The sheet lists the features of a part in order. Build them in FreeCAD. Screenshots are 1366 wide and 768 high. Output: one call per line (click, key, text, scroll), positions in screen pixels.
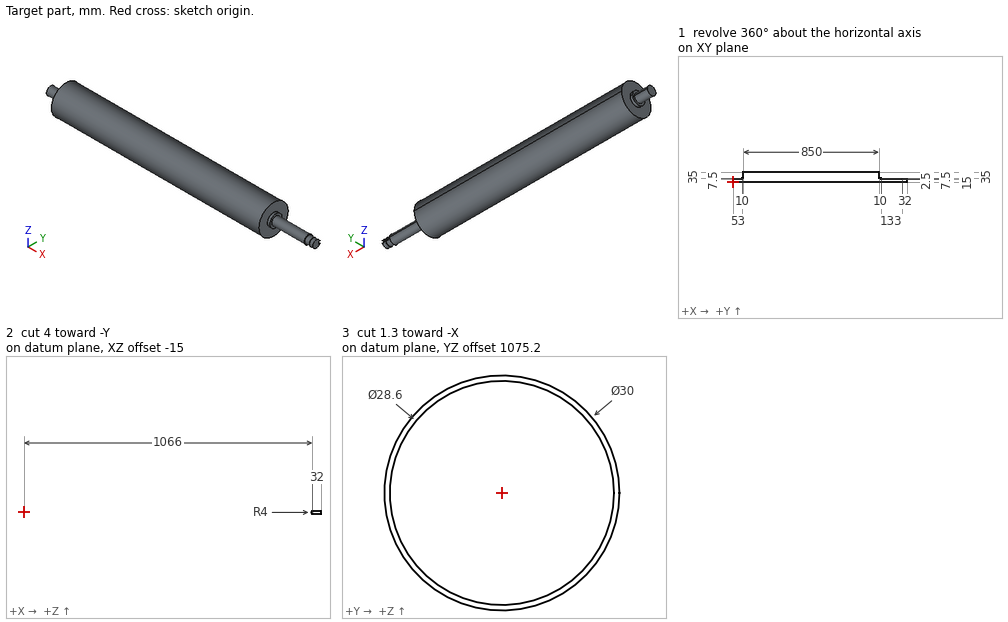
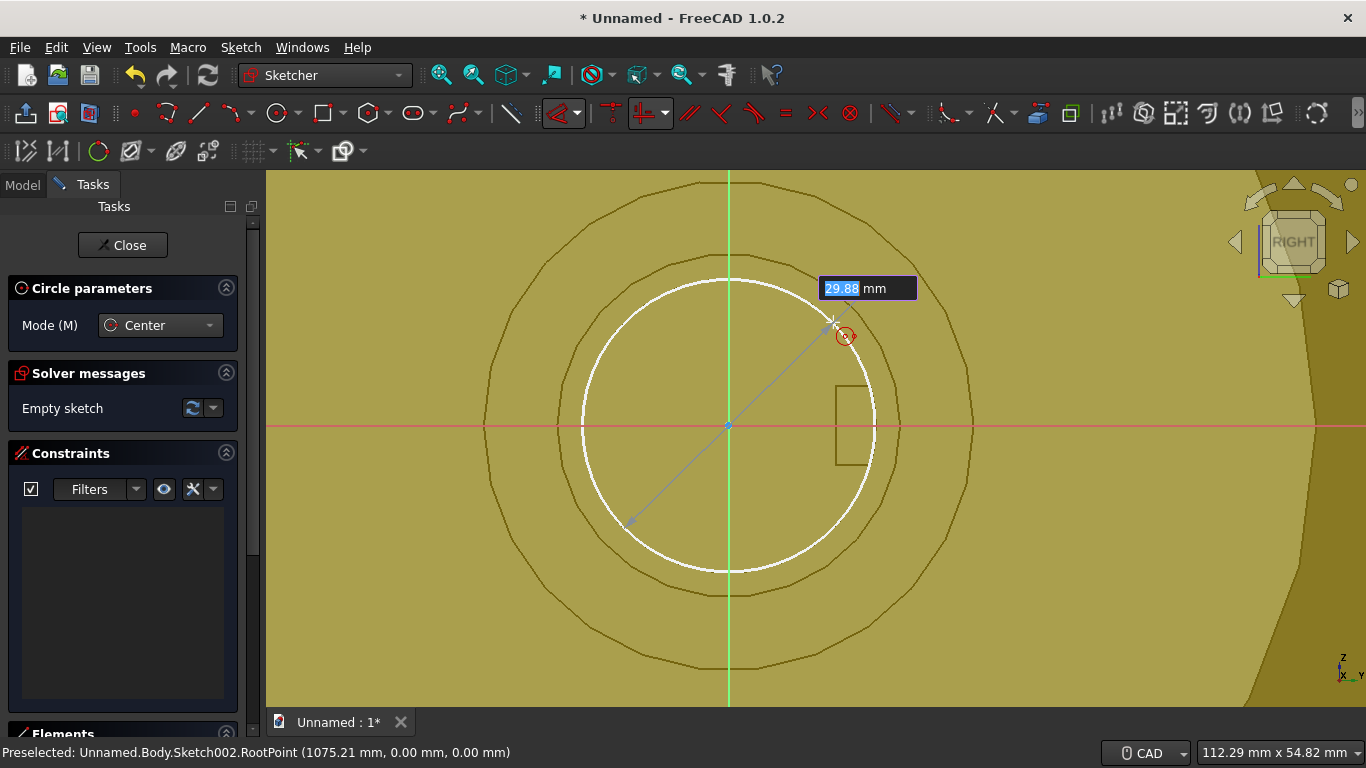
text(30)
key(Return)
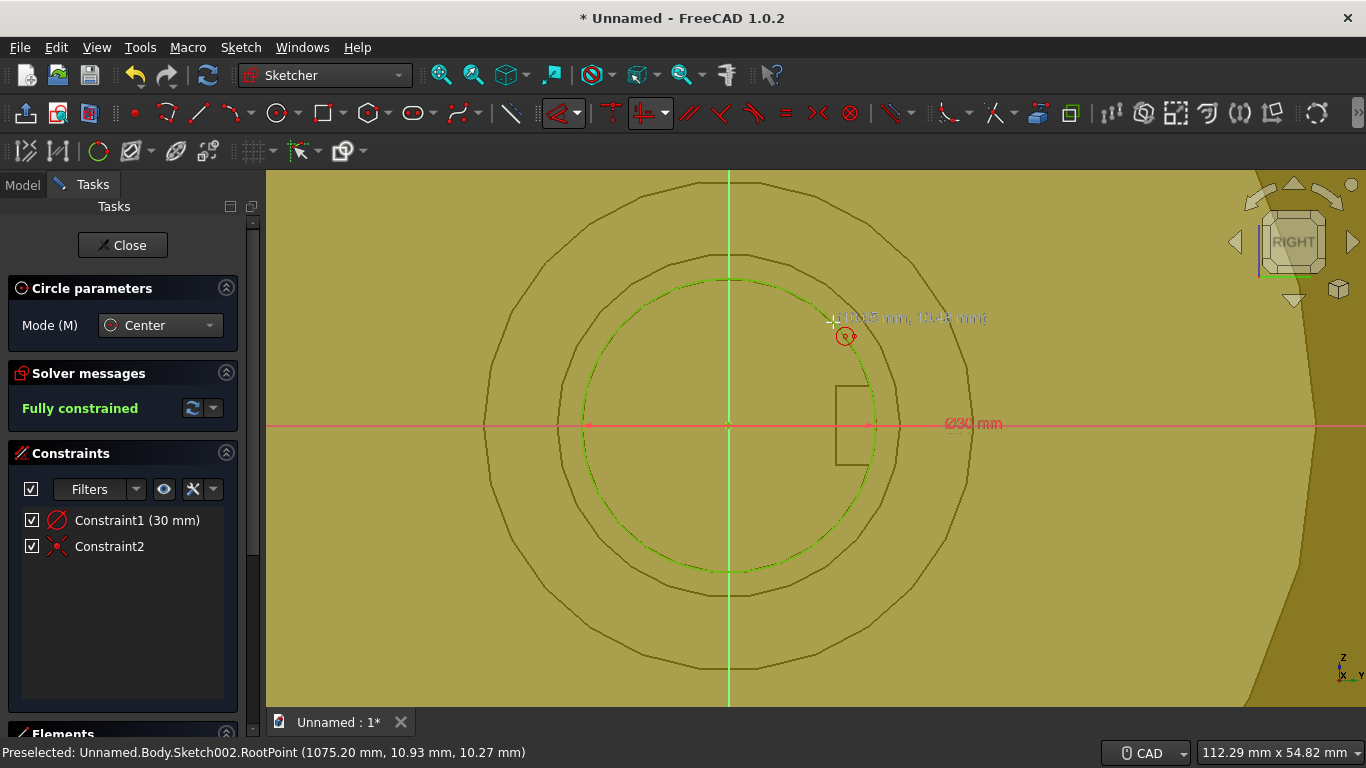
click(729, 426)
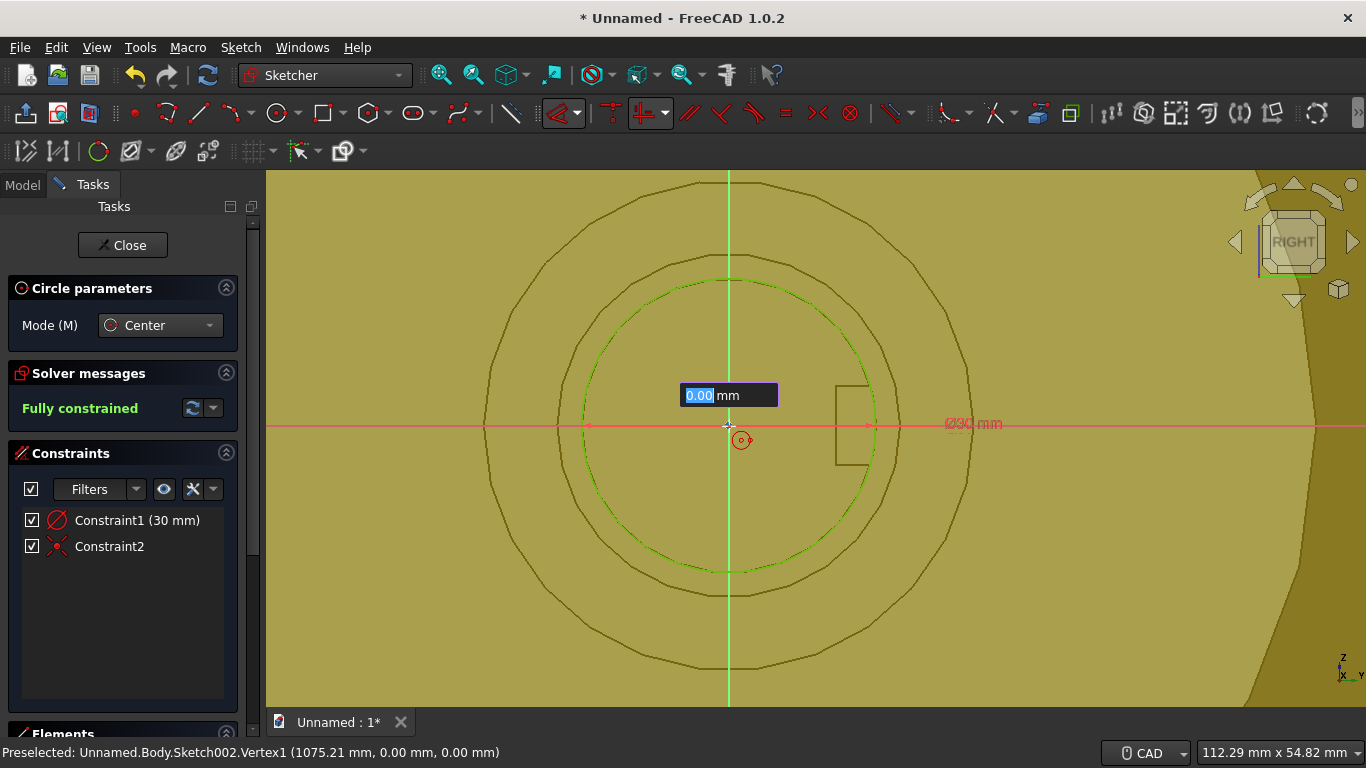
scroll(777, 294, up, 5)
move(775, 294)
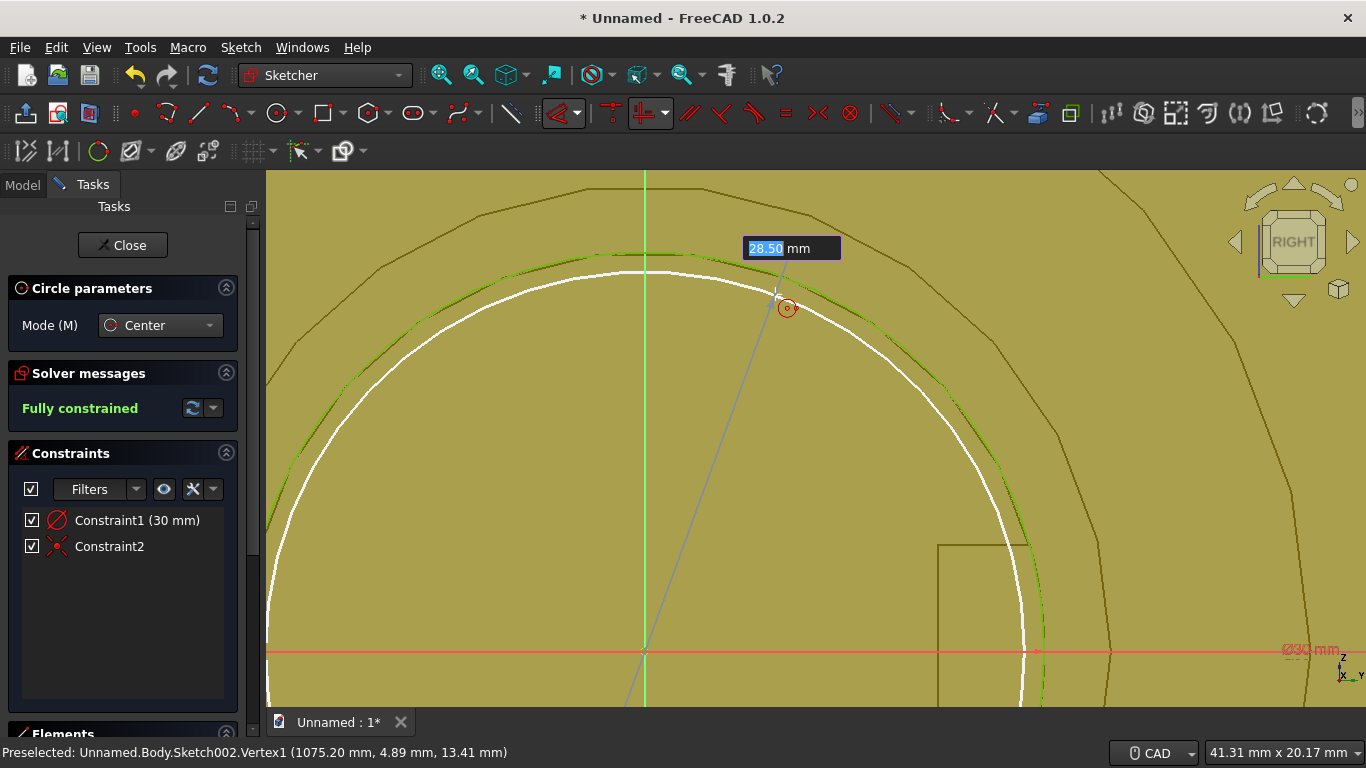
text(28.6)
key(Return)
key(Escape)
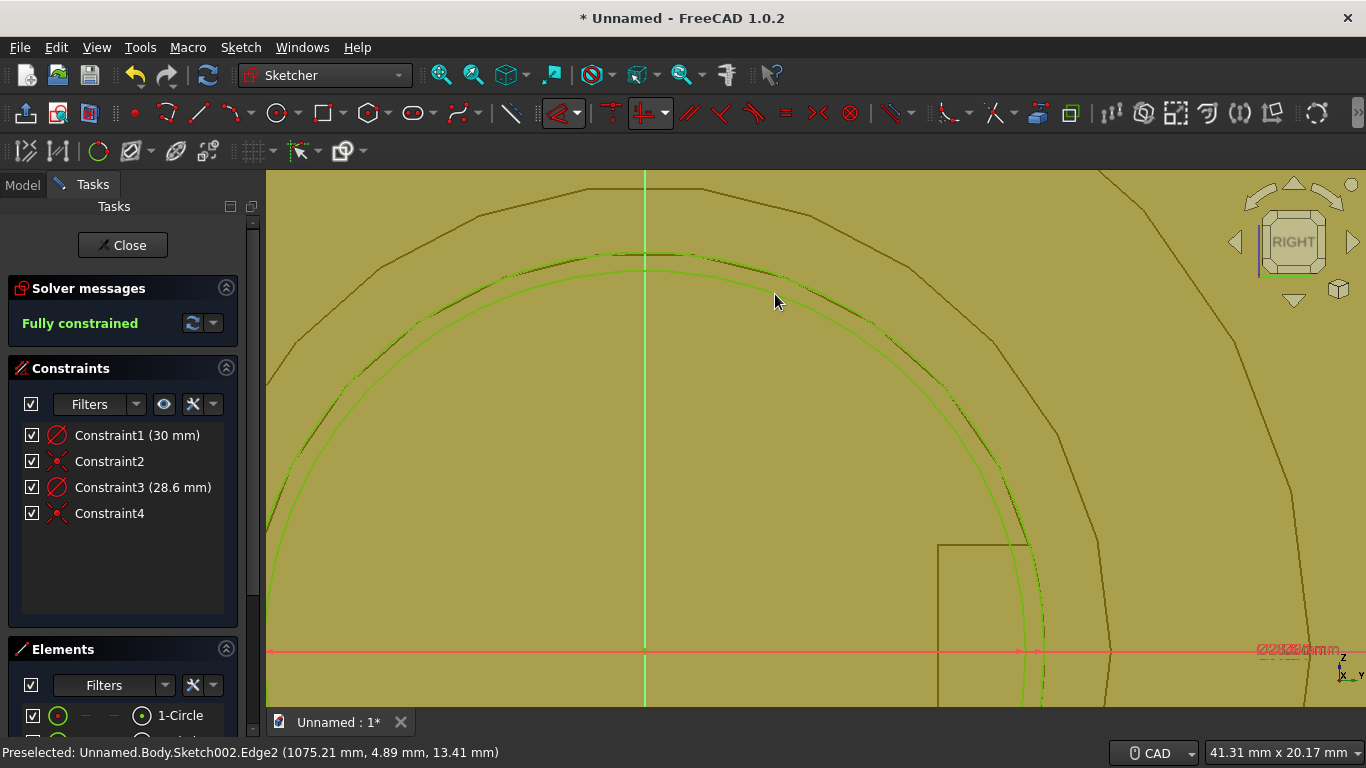
click(123, 245)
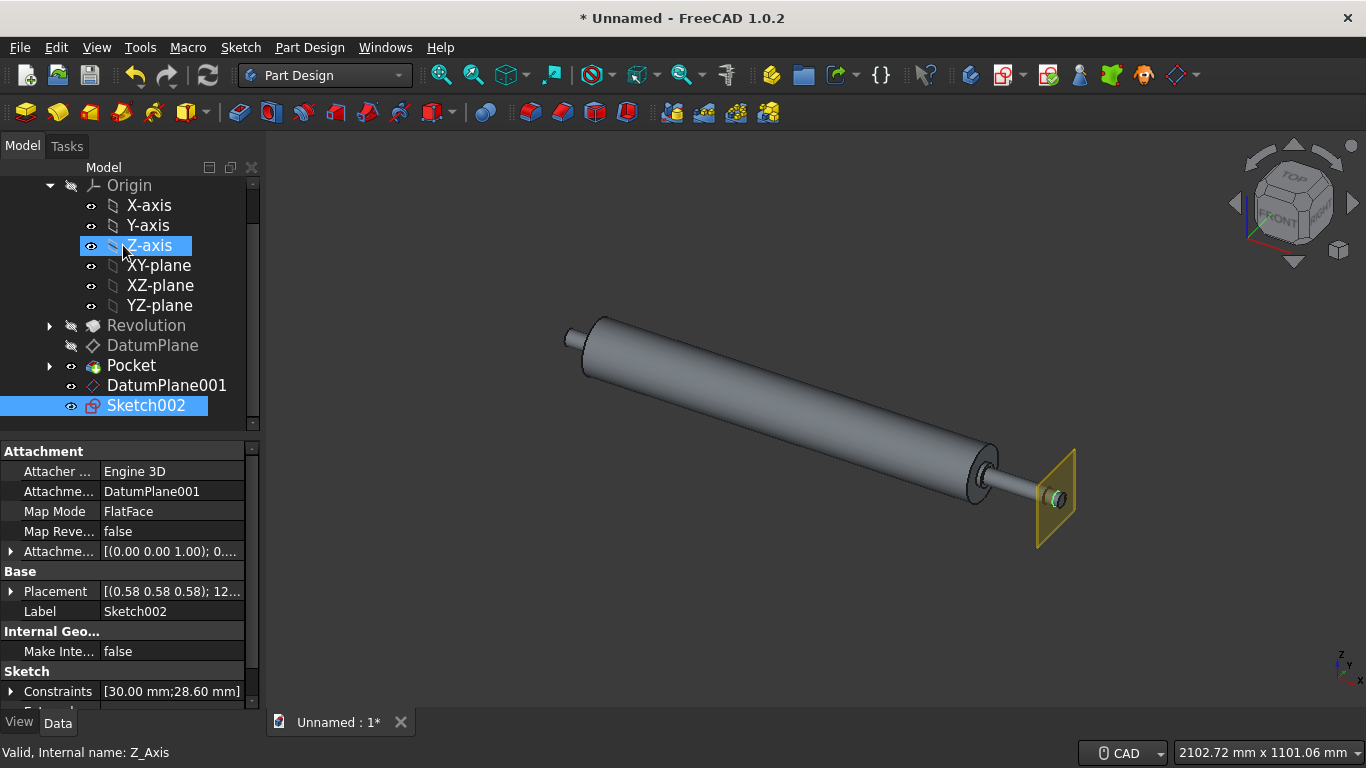
click(240, 112)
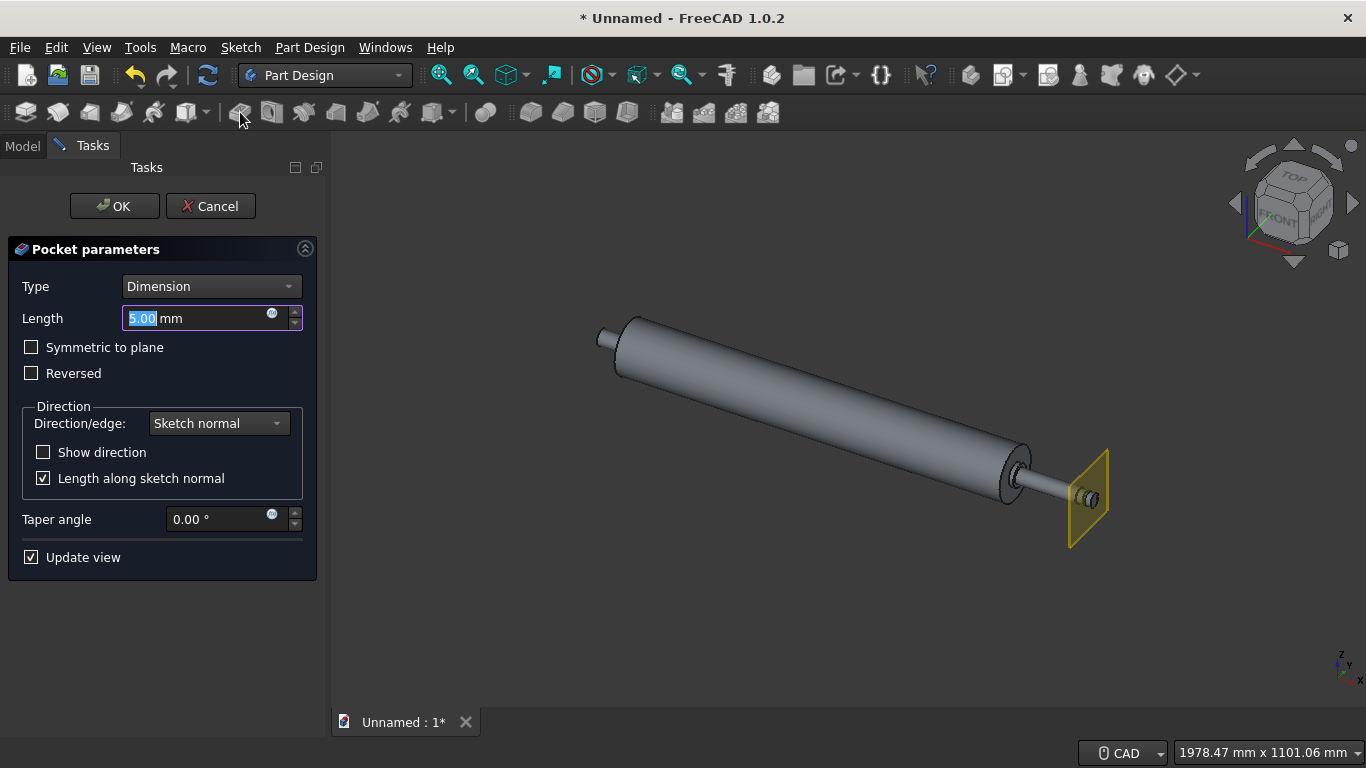
text(1.3)
key(Tab)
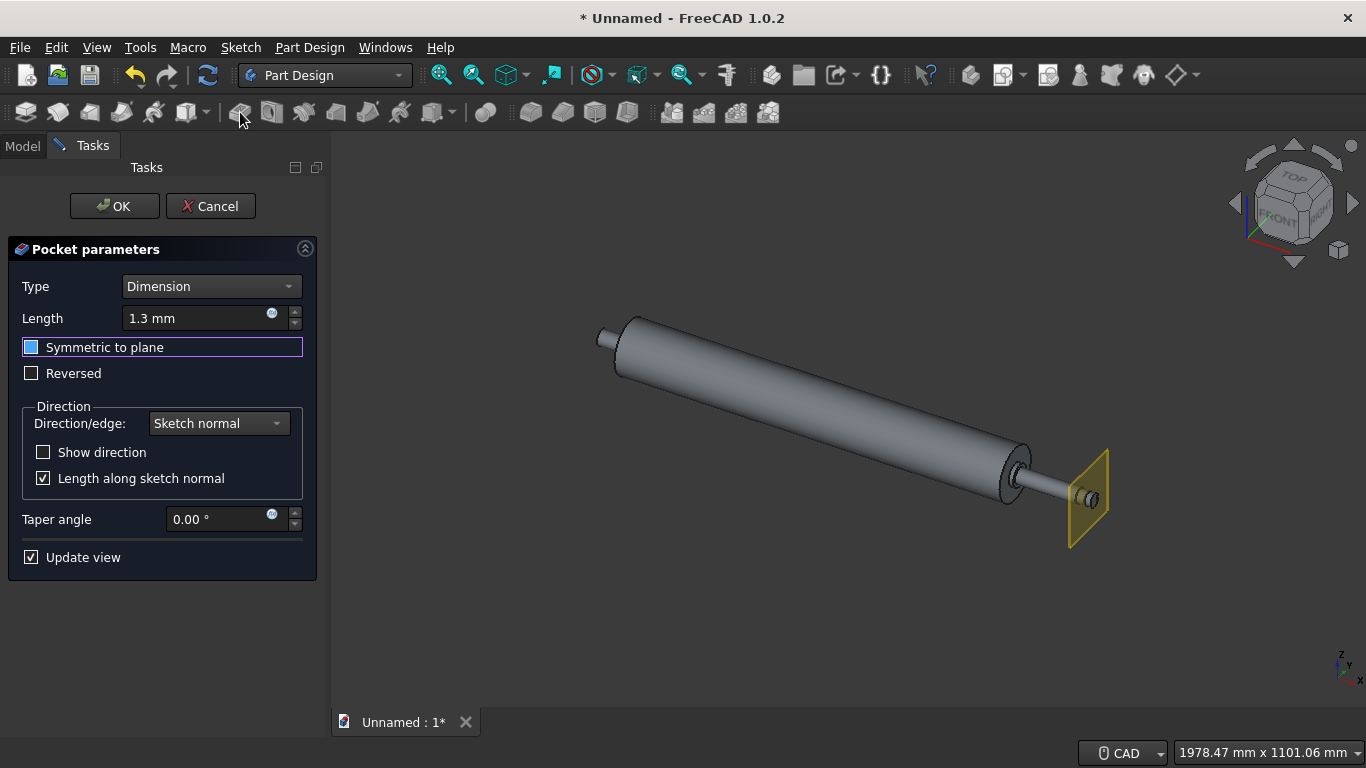
click(115, 206)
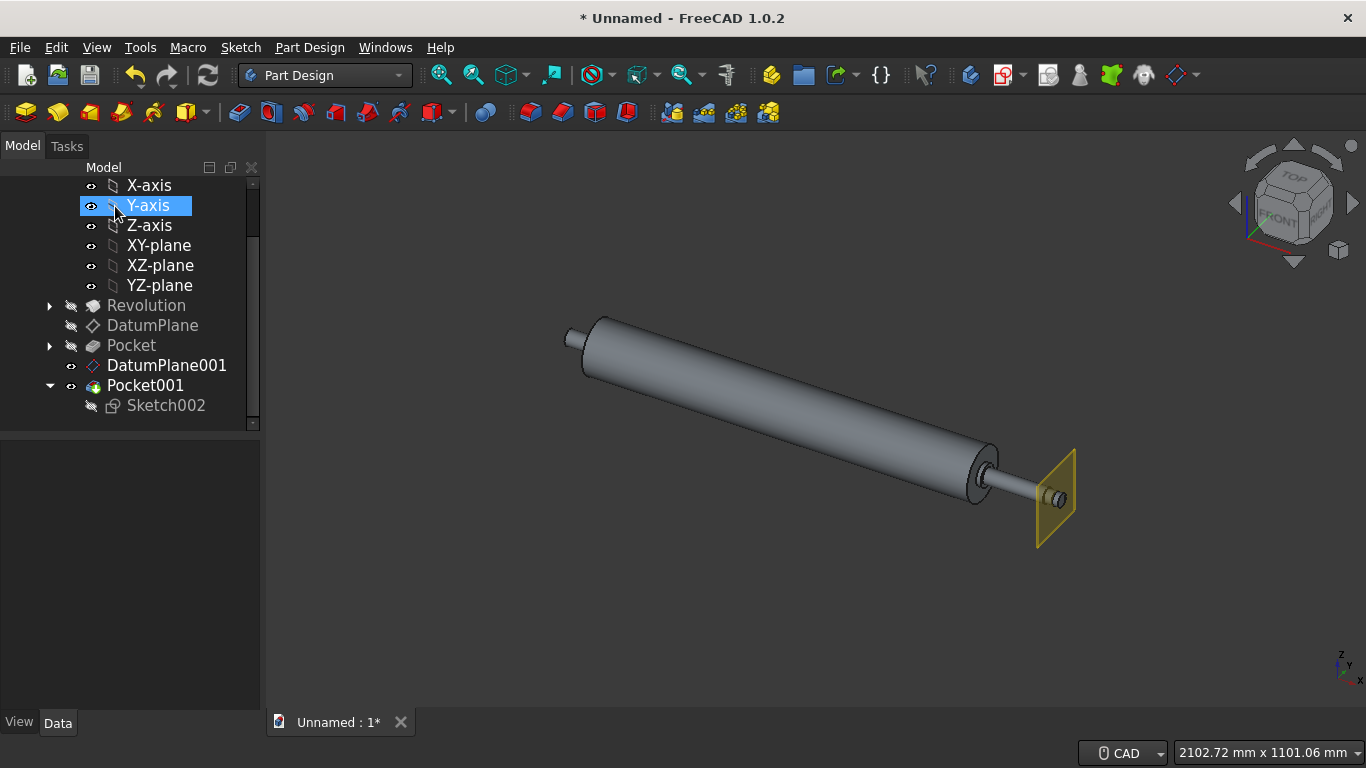
click(116, 366)
key(space)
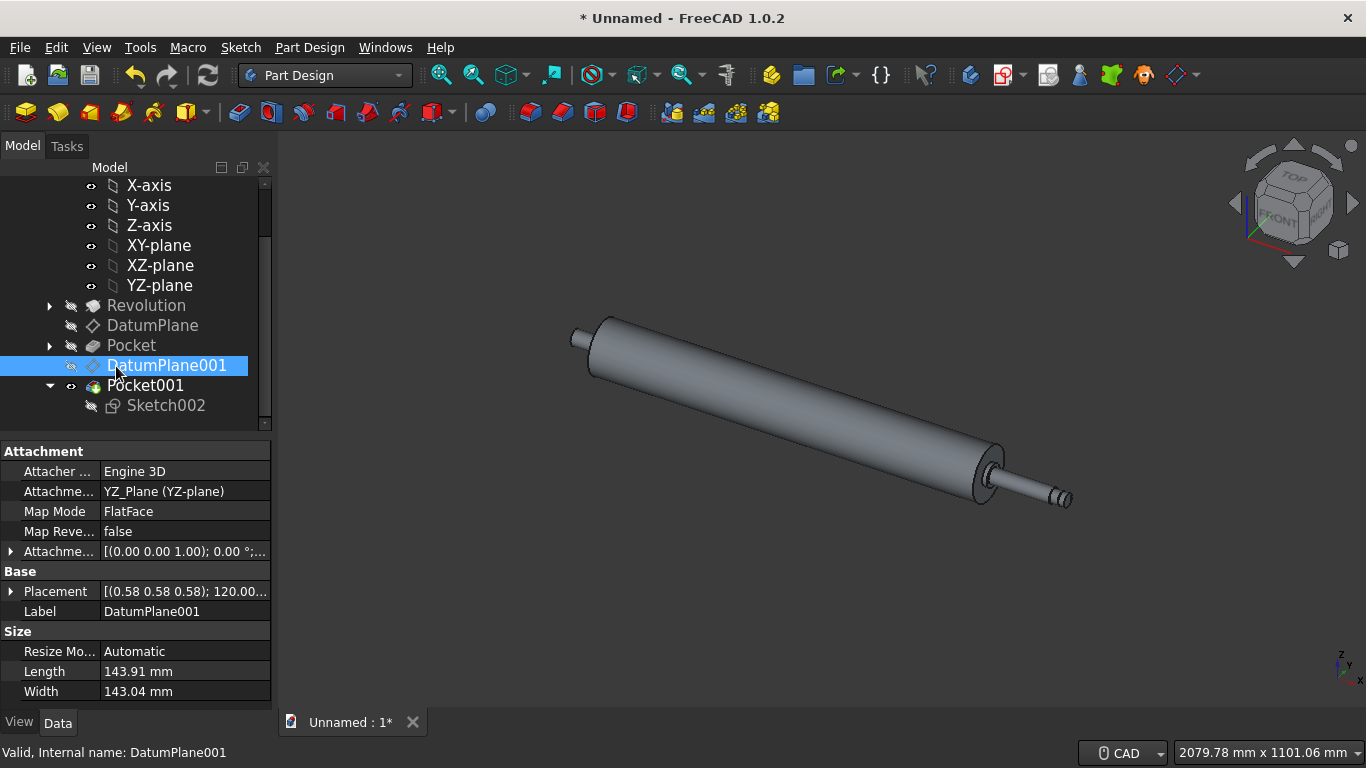
key(0)